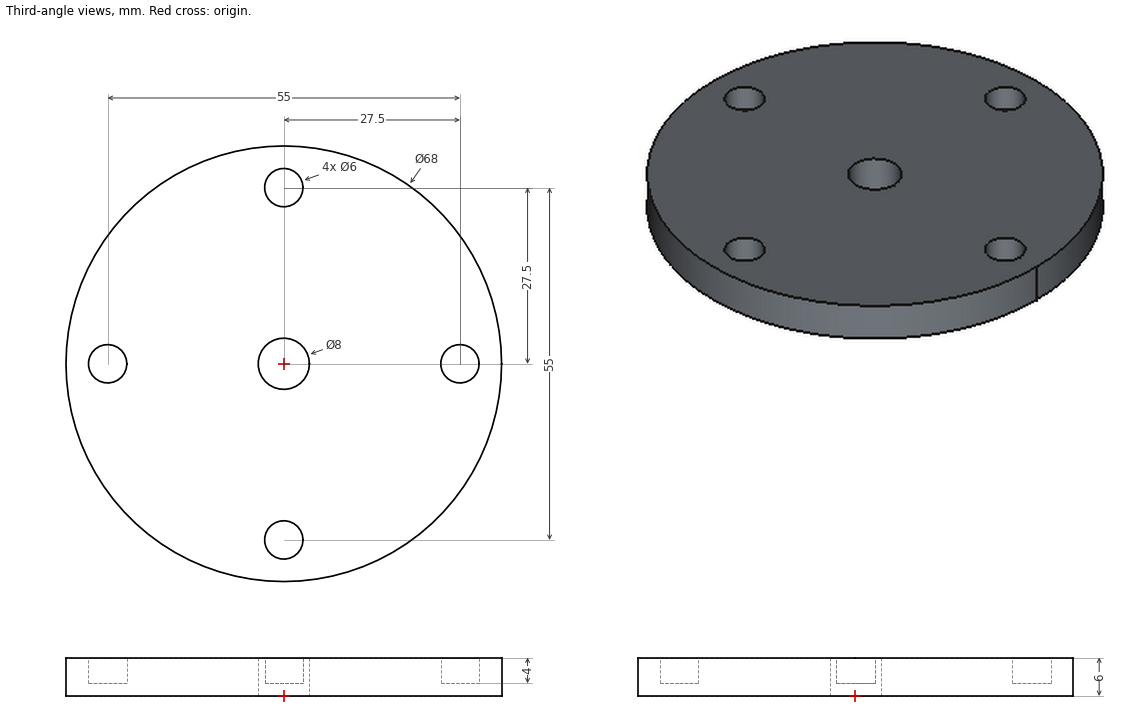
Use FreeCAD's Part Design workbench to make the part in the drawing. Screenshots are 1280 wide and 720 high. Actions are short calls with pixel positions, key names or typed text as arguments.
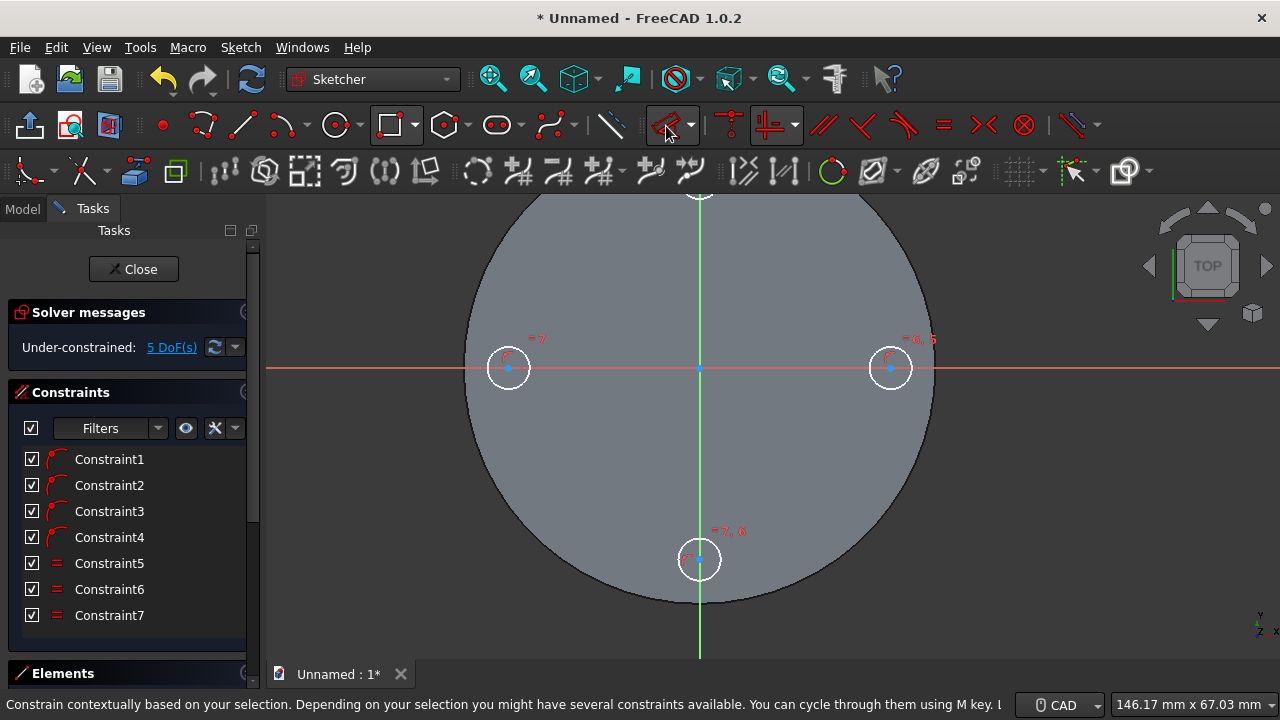
scroll(715, 545, down, 2)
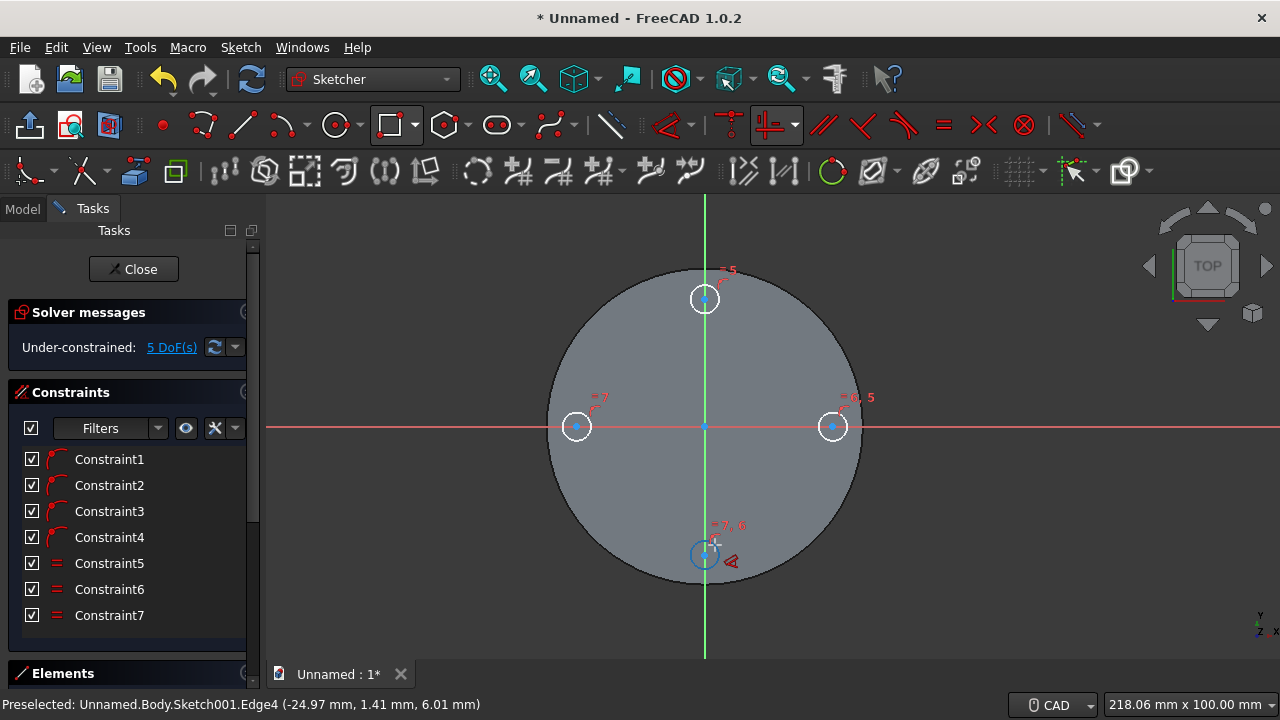
scroll(715, 289, up, 2)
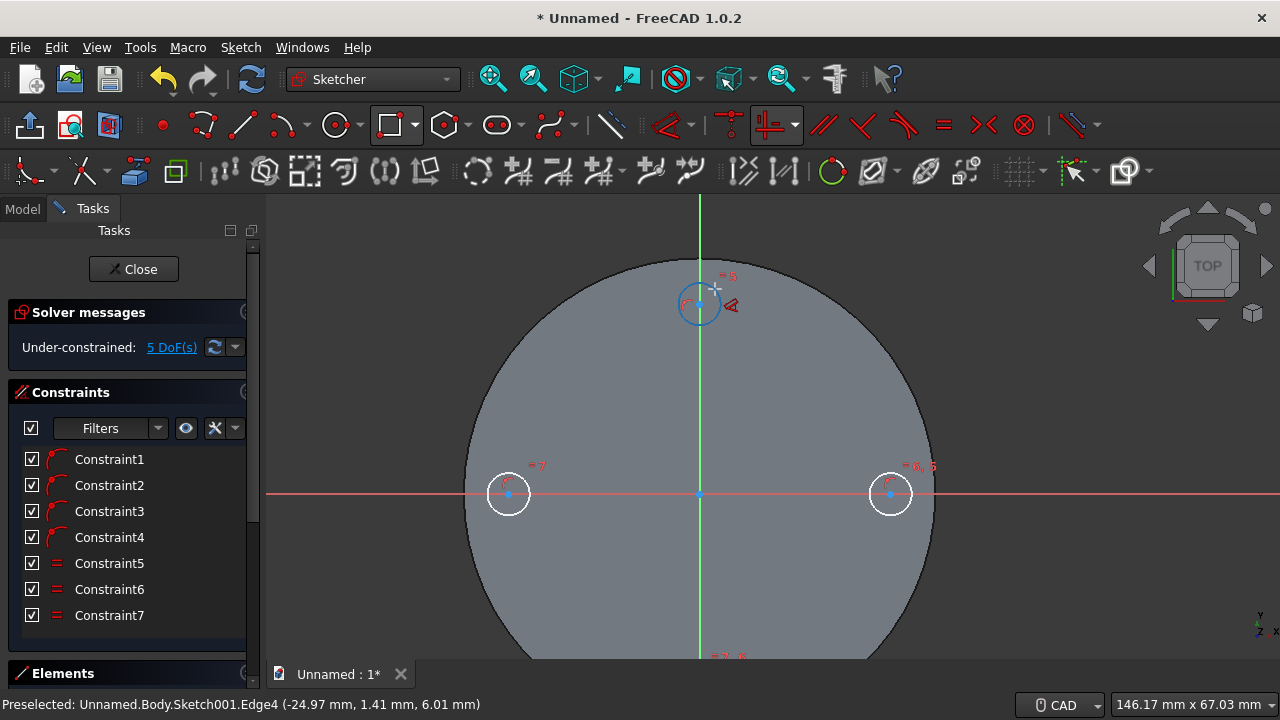
click(714, 289)
click(736, 266)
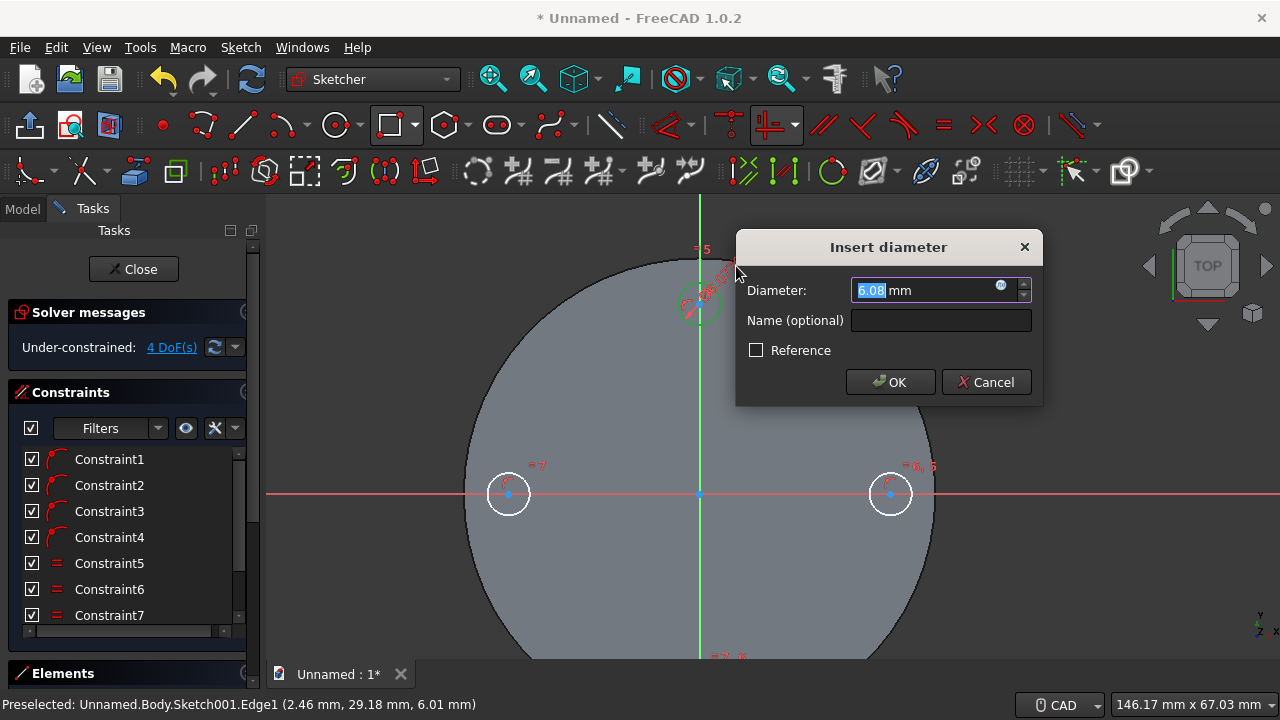
text(6)
key(Return)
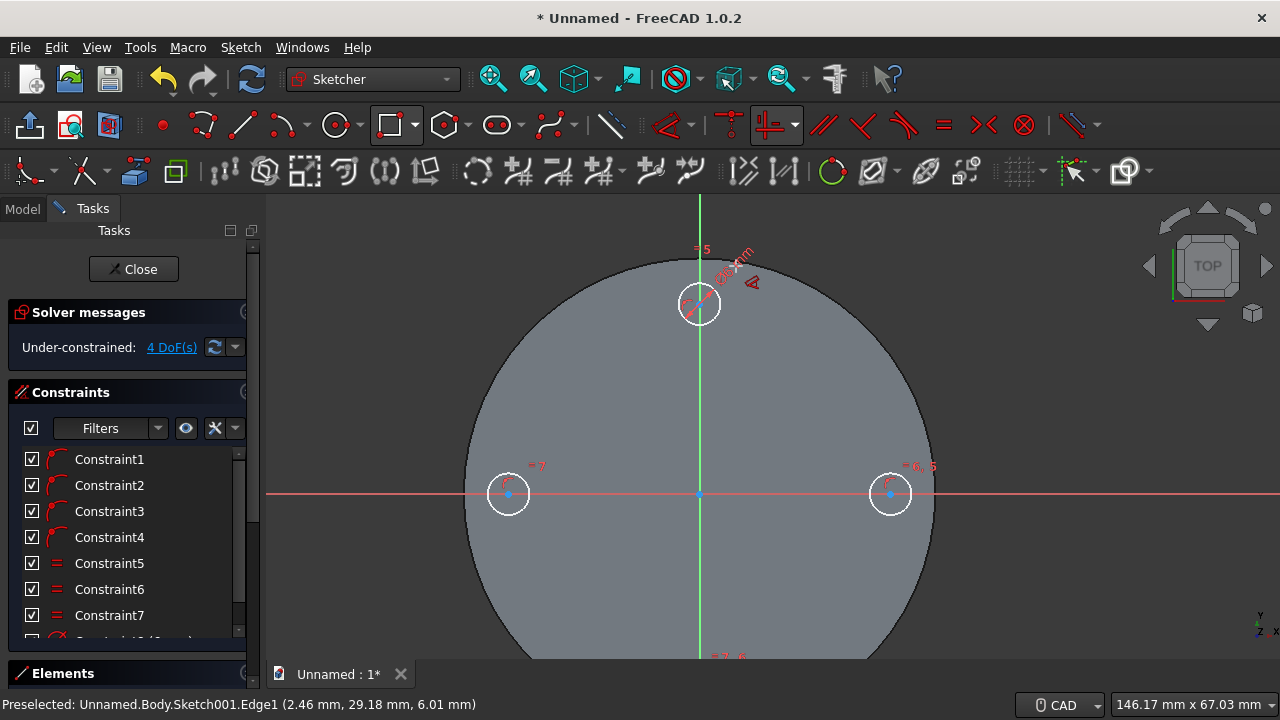
click(700, 304)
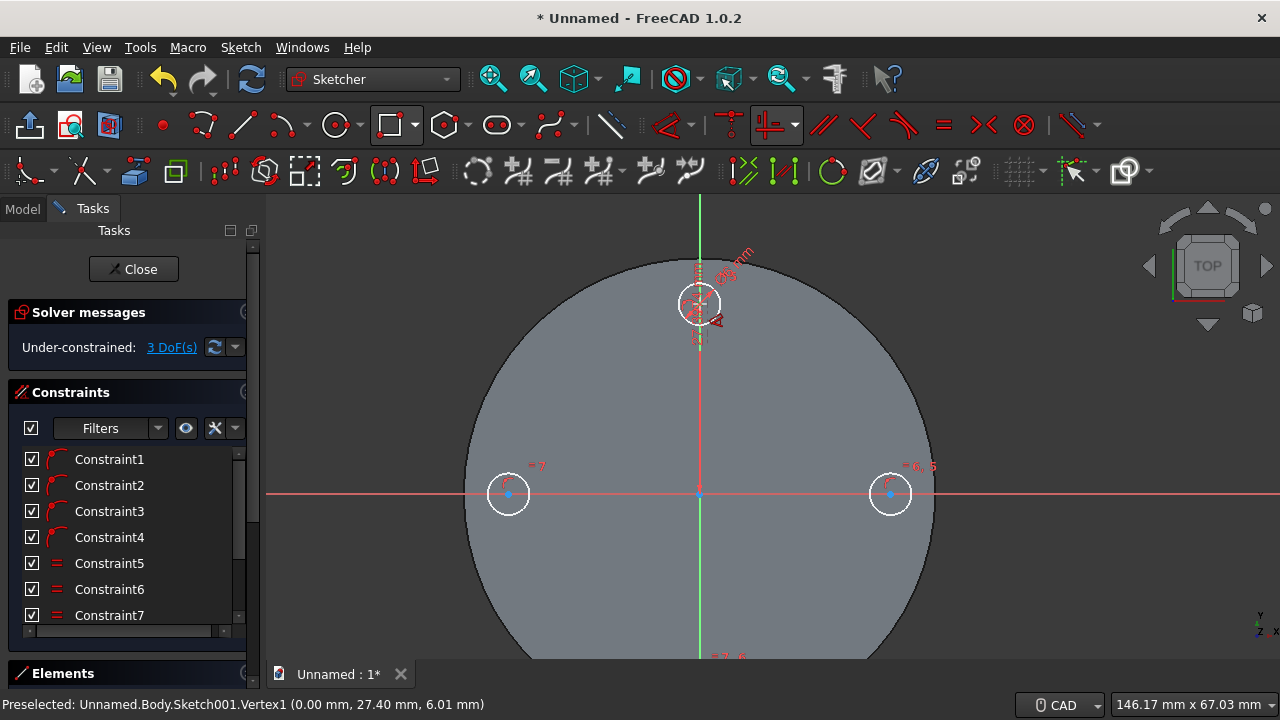
scroll(715, 289, down, 2)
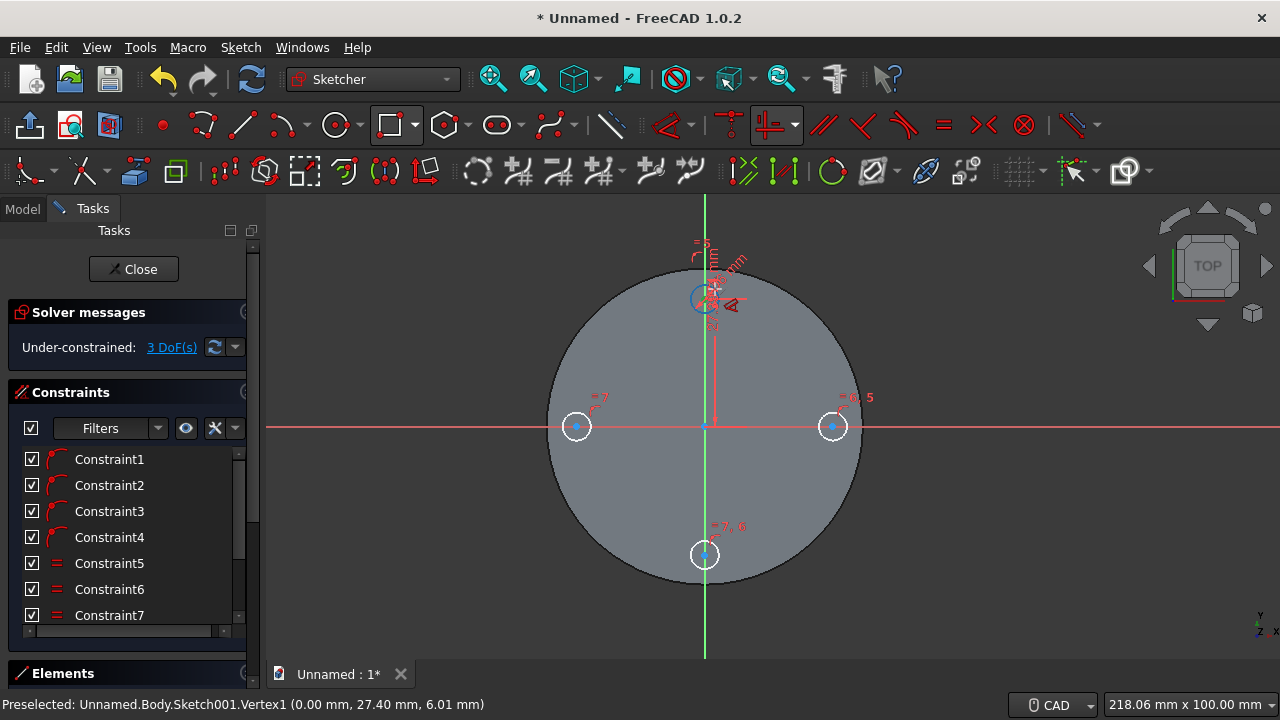
click(705, 555)
click(739, 368)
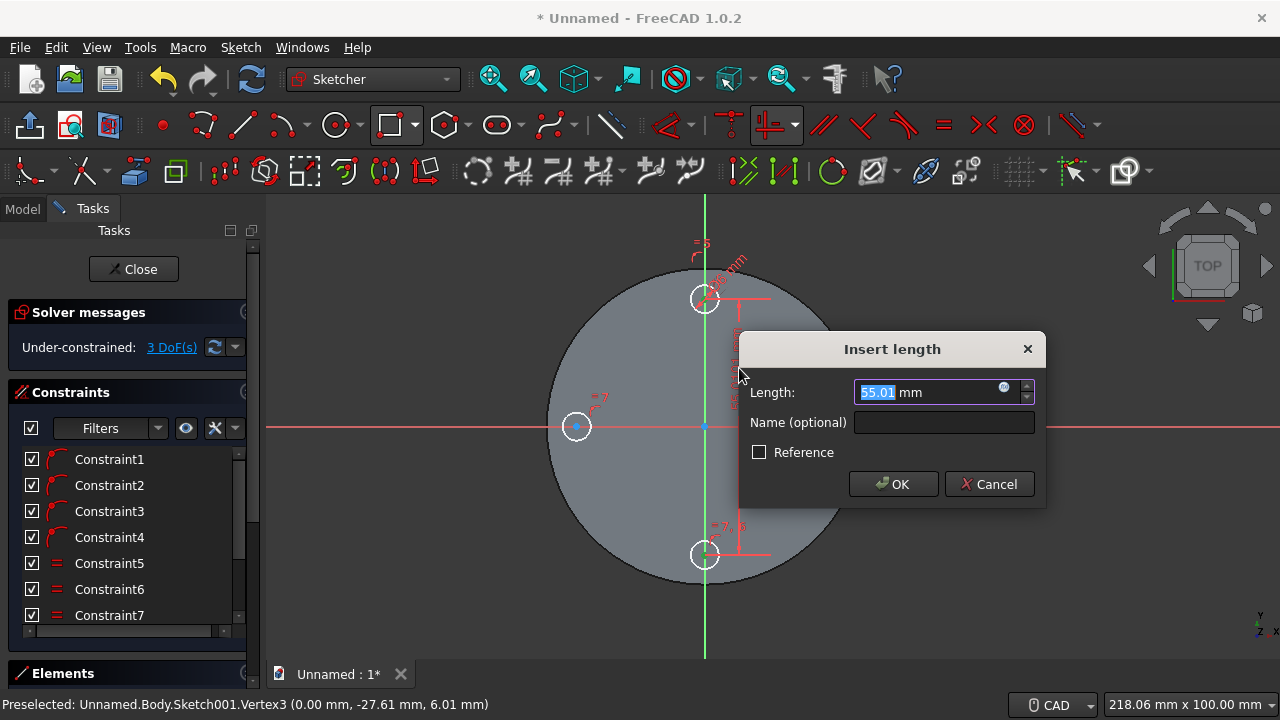
text(55)
key(Return)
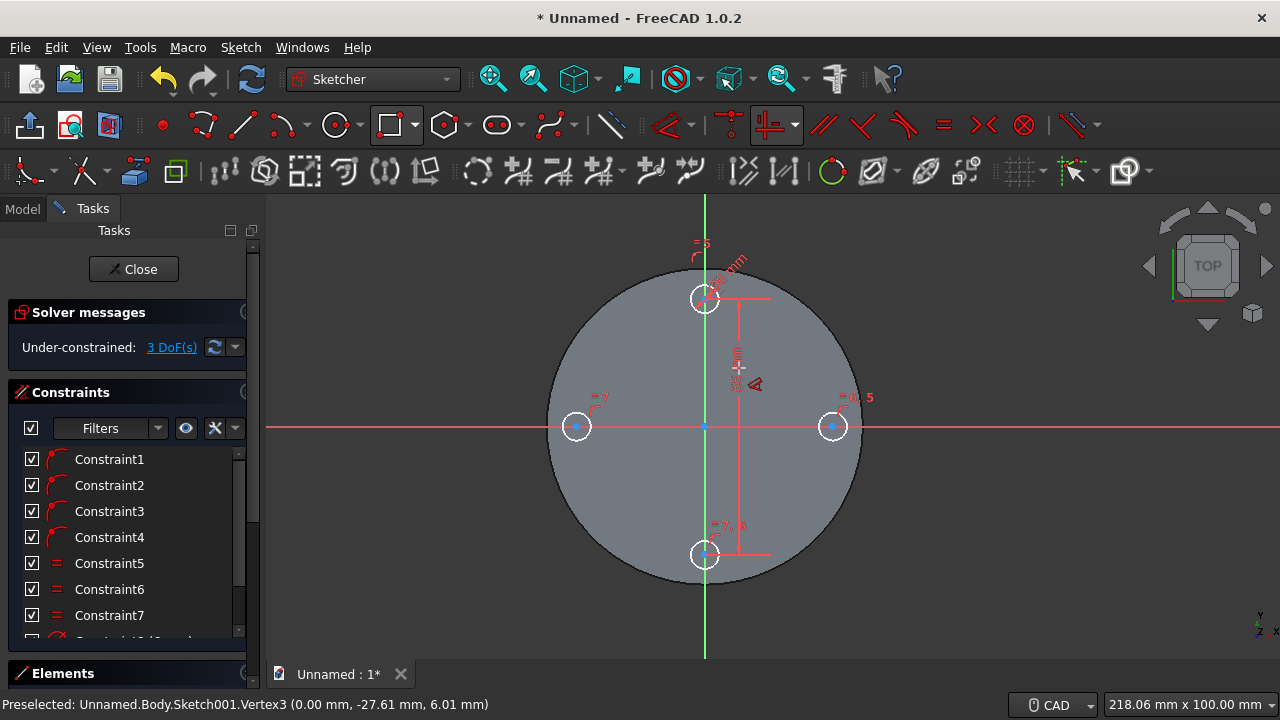
click(833, 427)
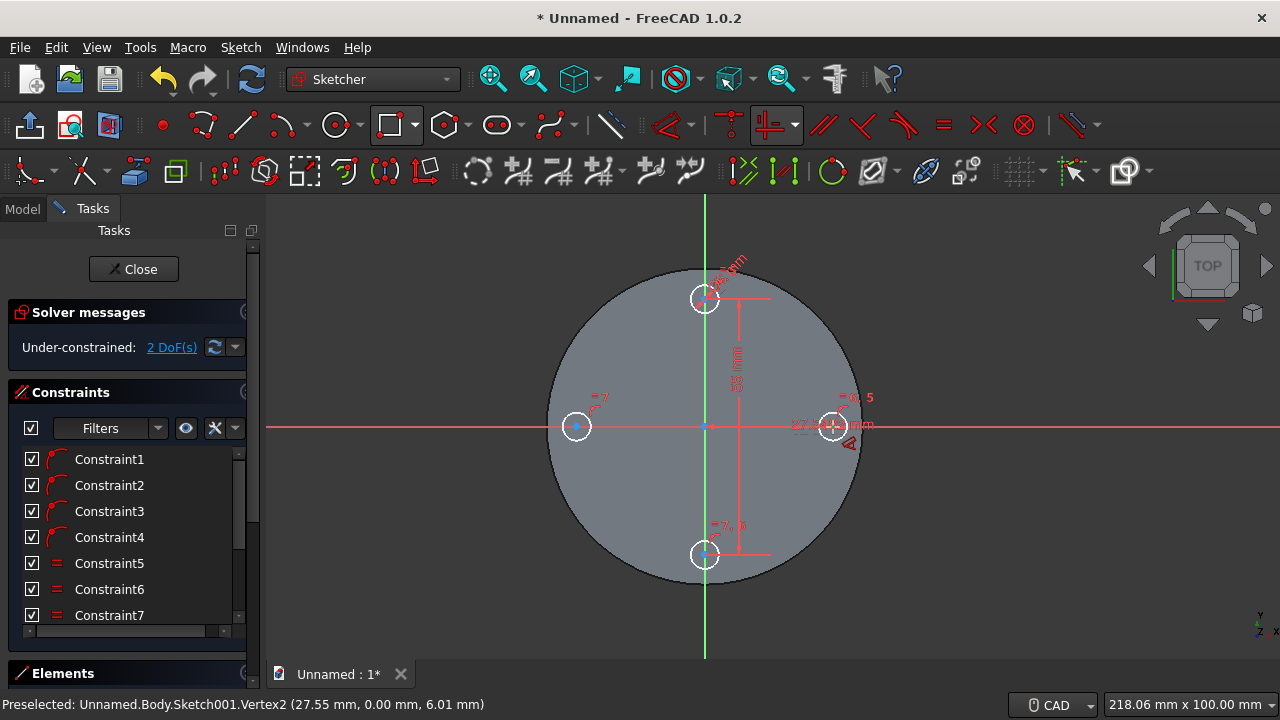
click(577, 427)
click(646, 461)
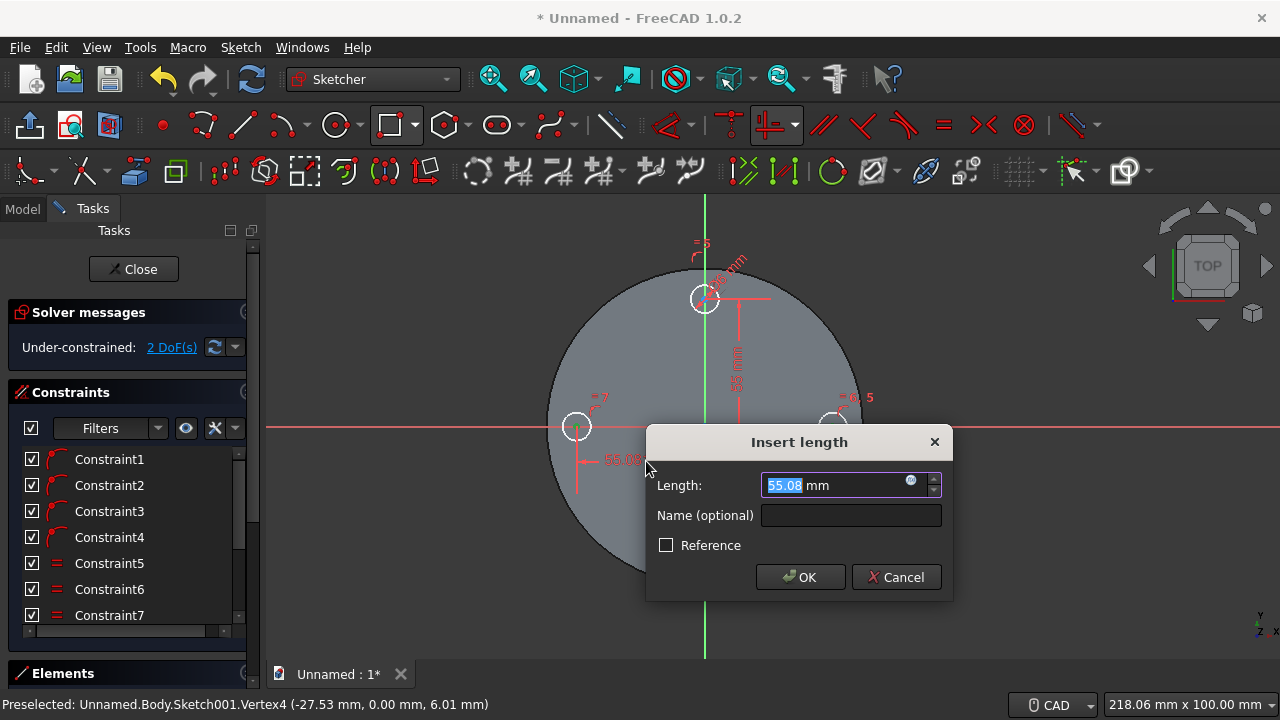
text(55)
key(Return)